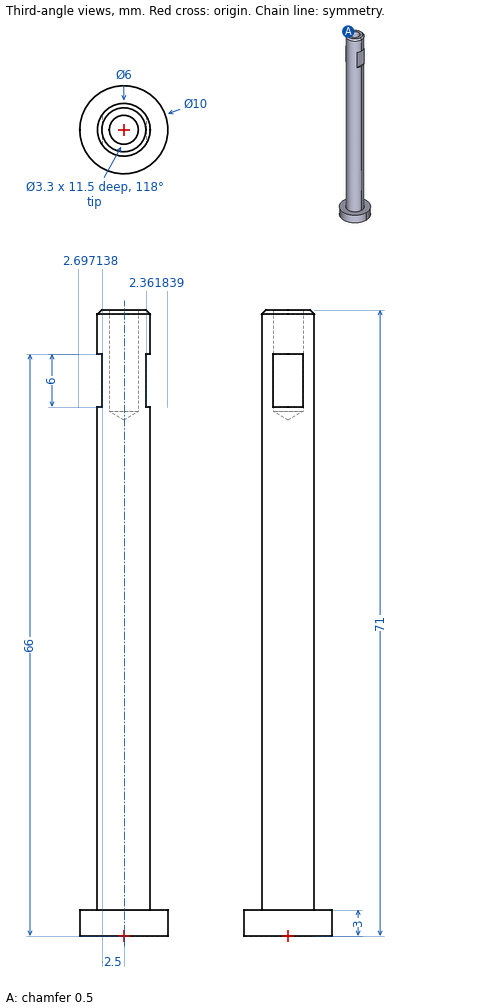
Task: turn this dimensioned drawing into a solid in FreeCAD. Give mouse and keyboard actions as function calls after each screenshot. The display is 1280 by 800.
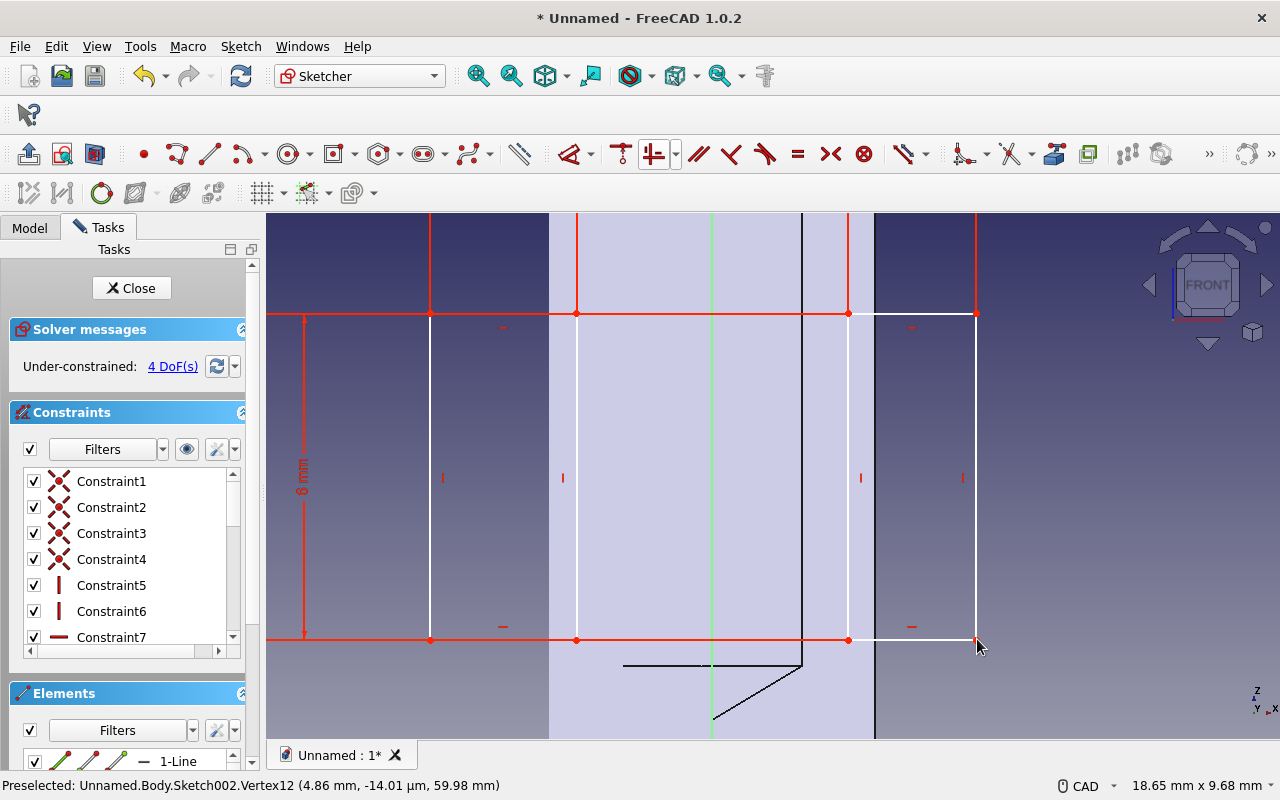
click(577, 314)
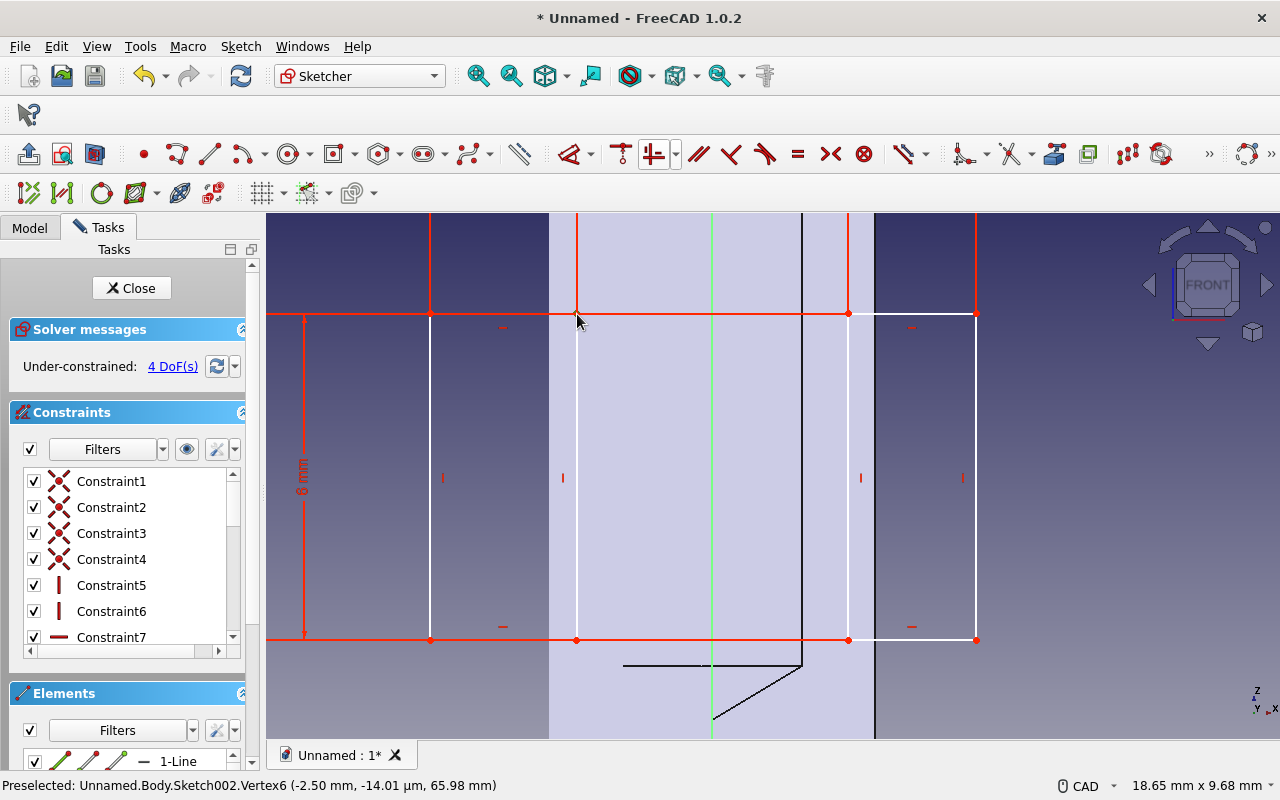
click(848, 314)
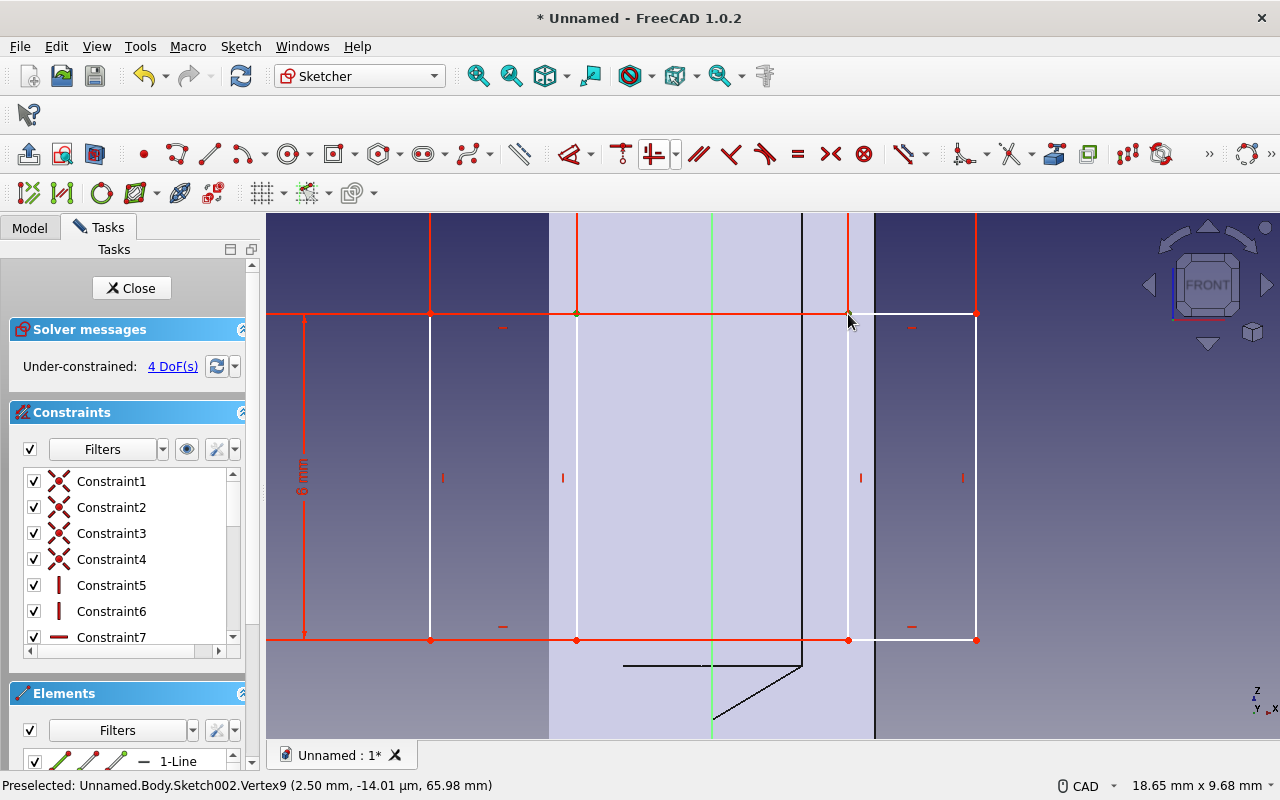
click(712, 677)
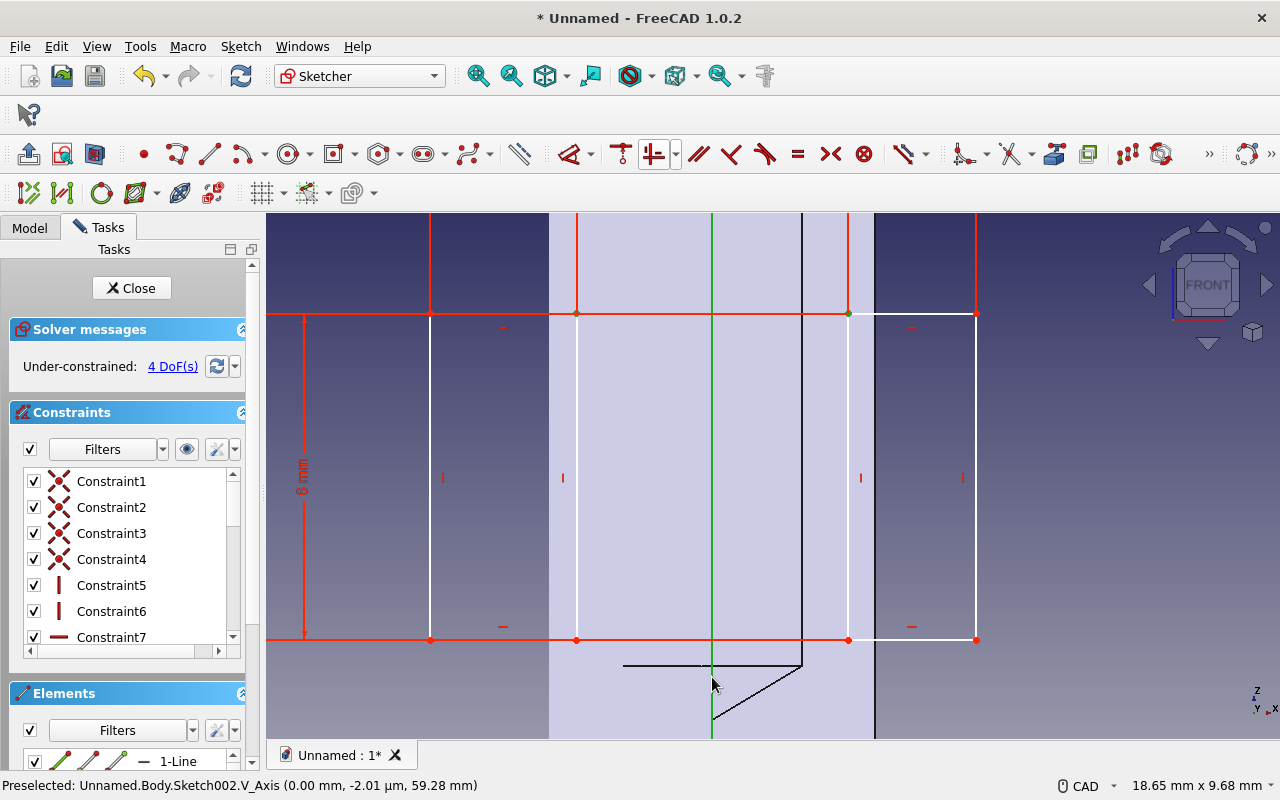
click(831, 154)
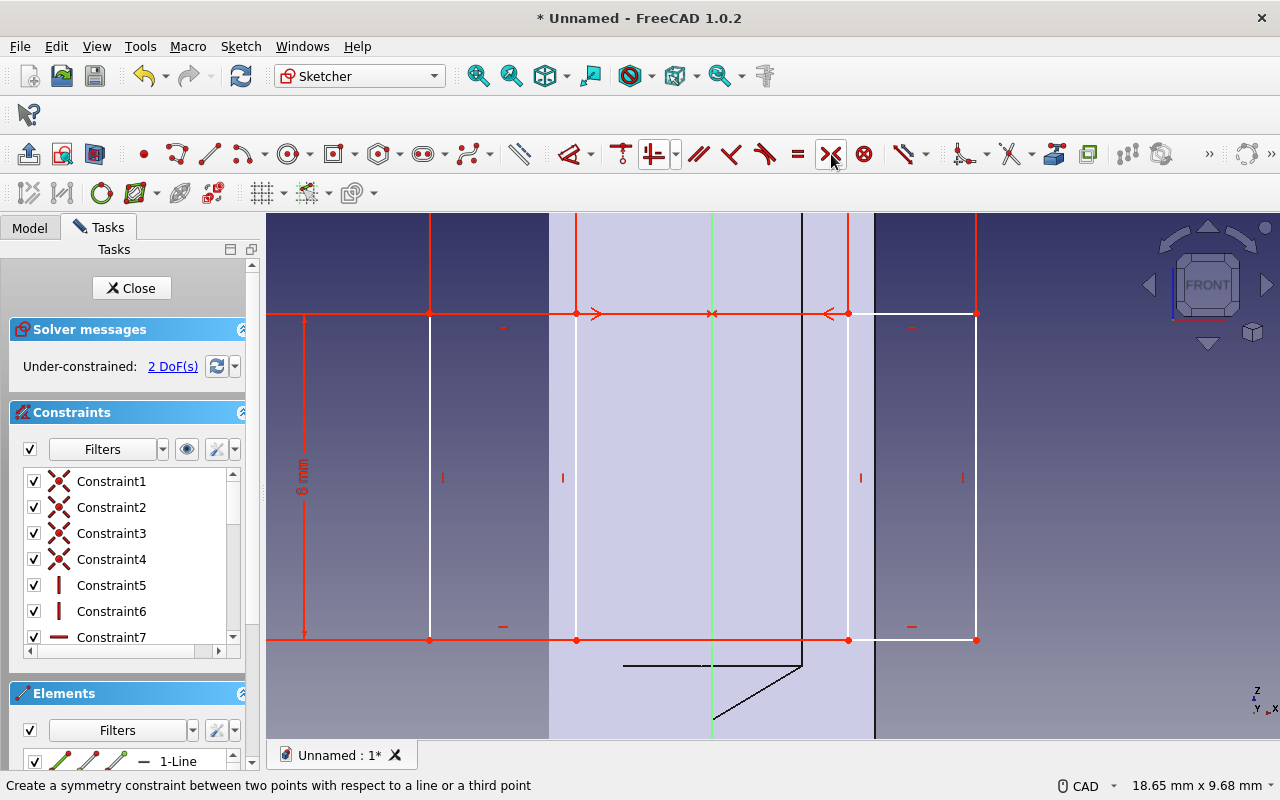
click(430, 314)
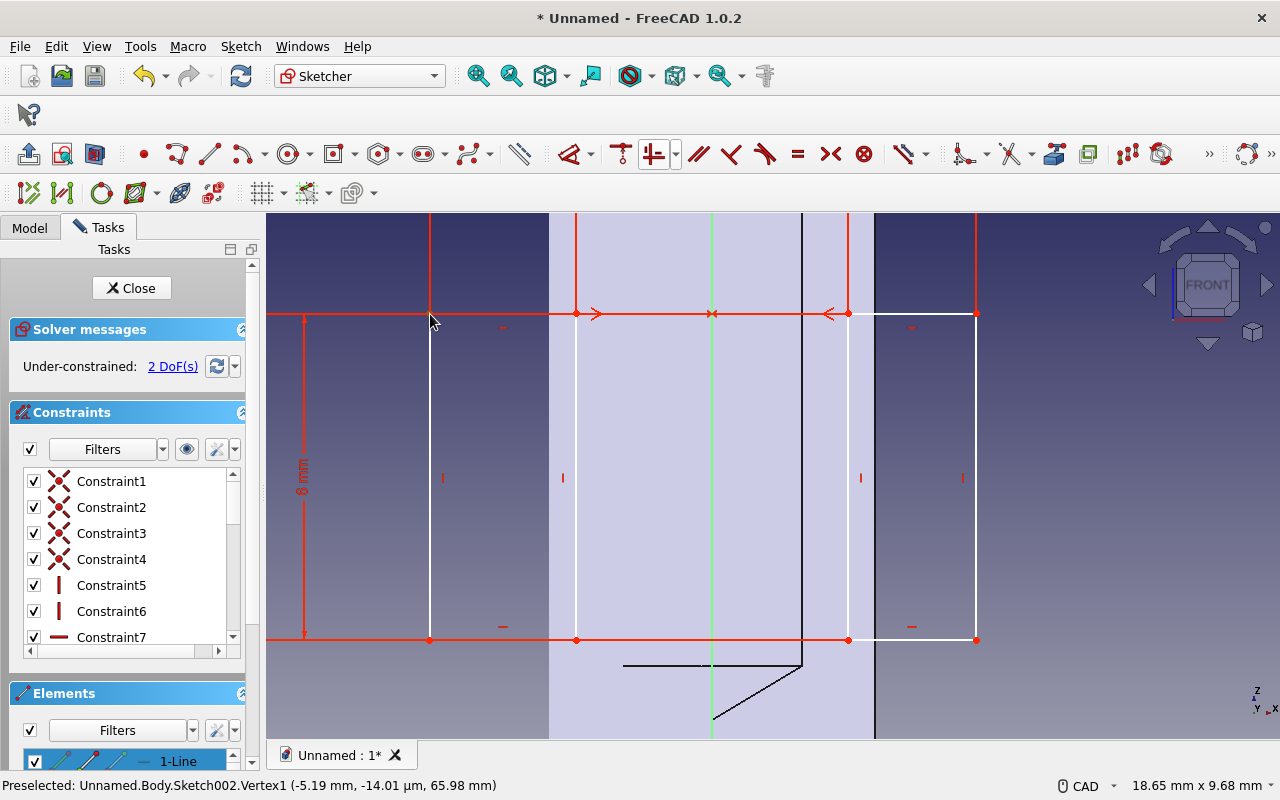
key(i)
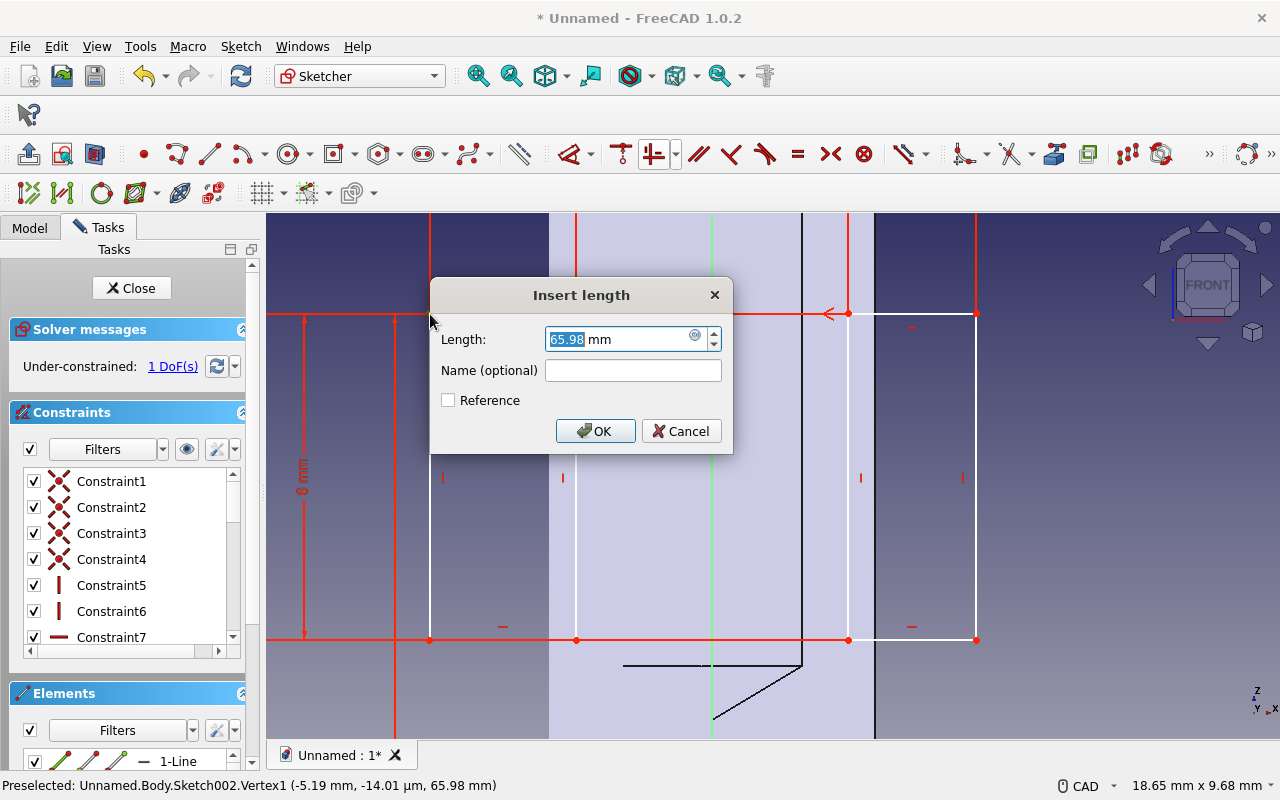
text(66)
key(Return)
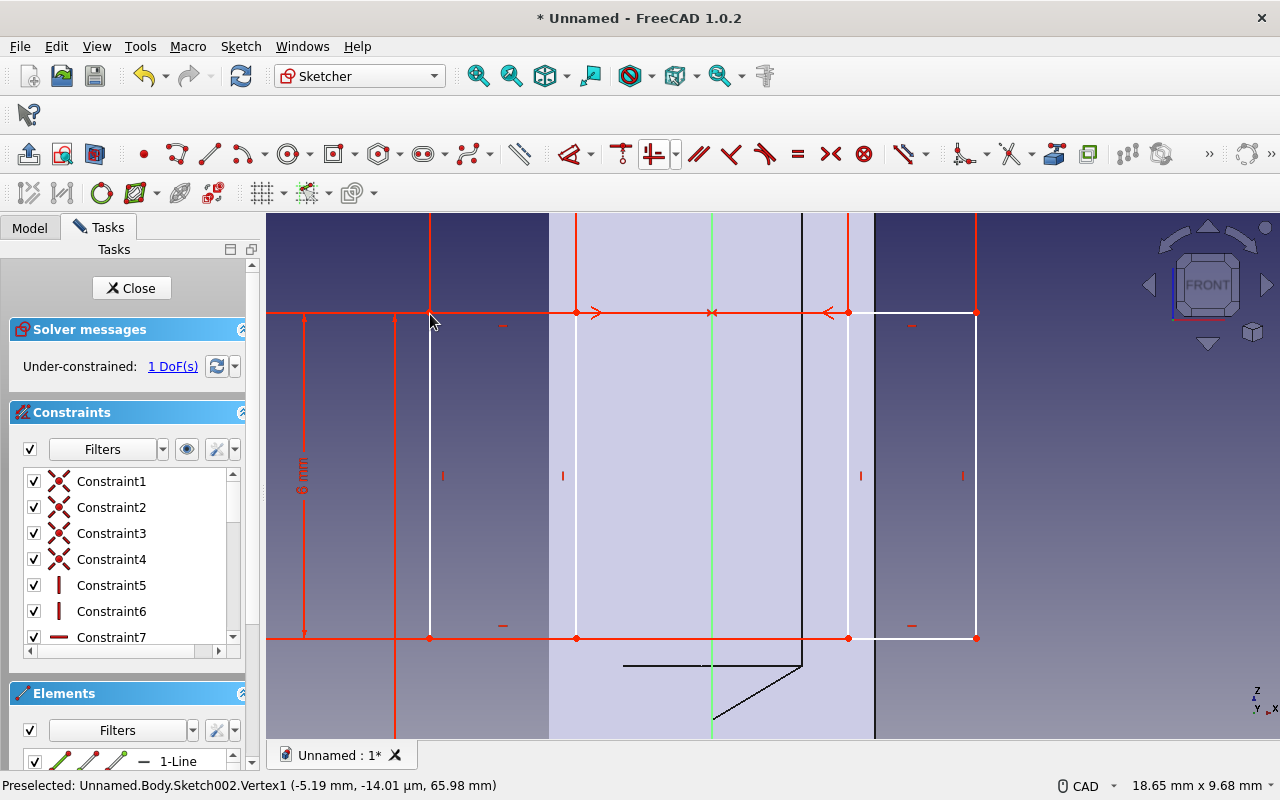
click(576, 639)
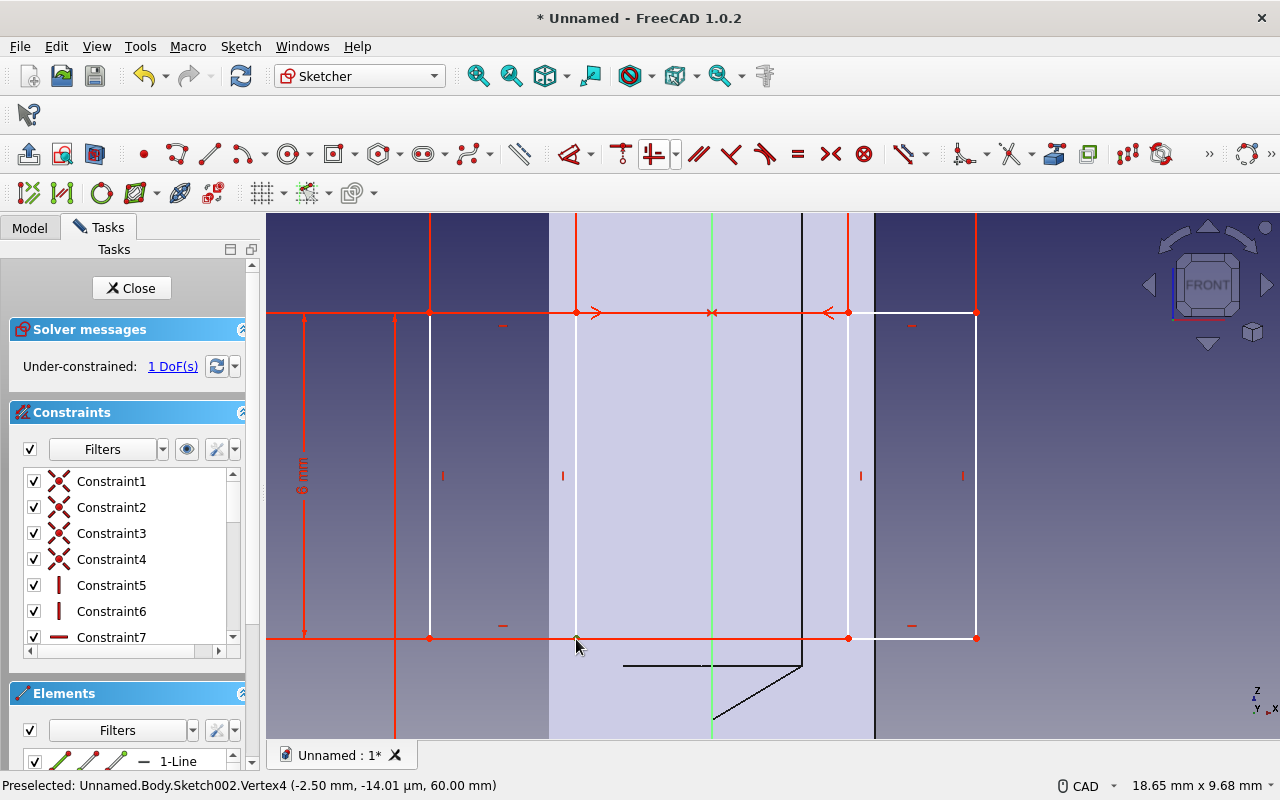
click(590, 154)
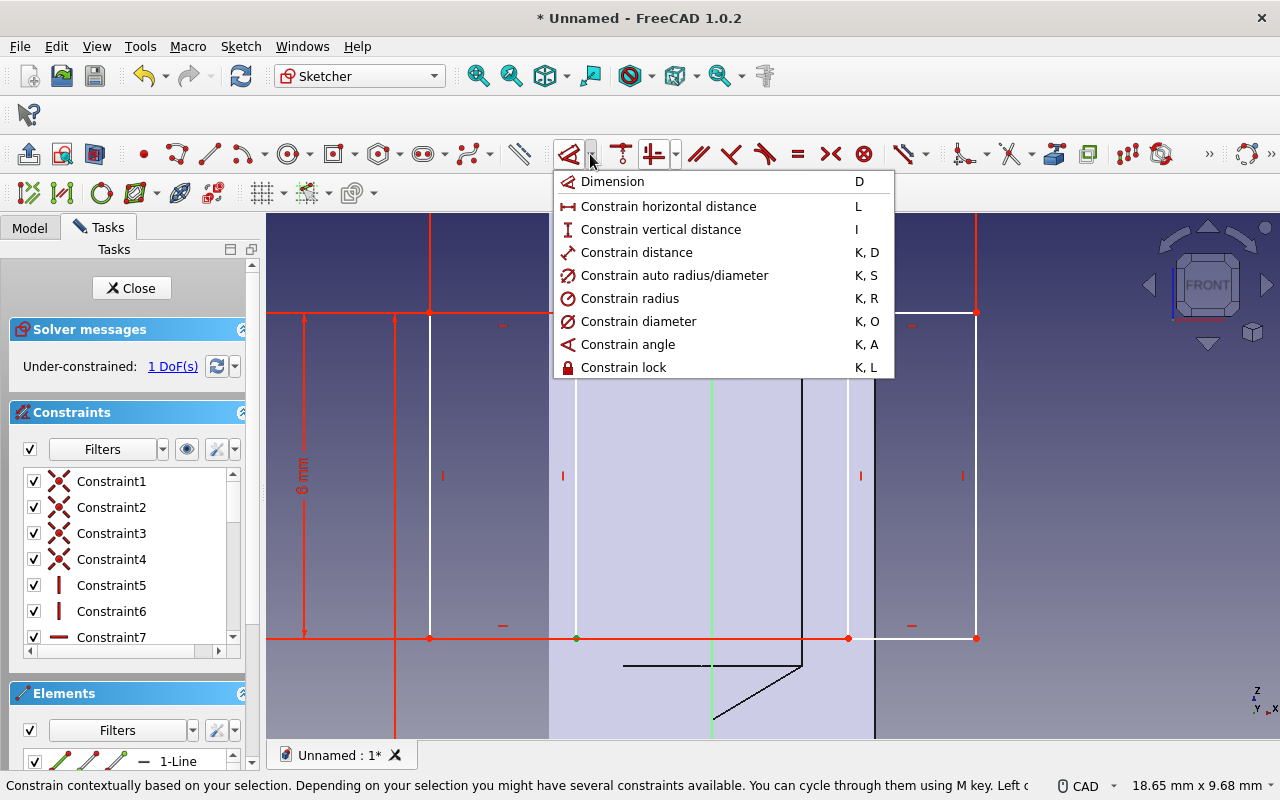
click(724, 206)